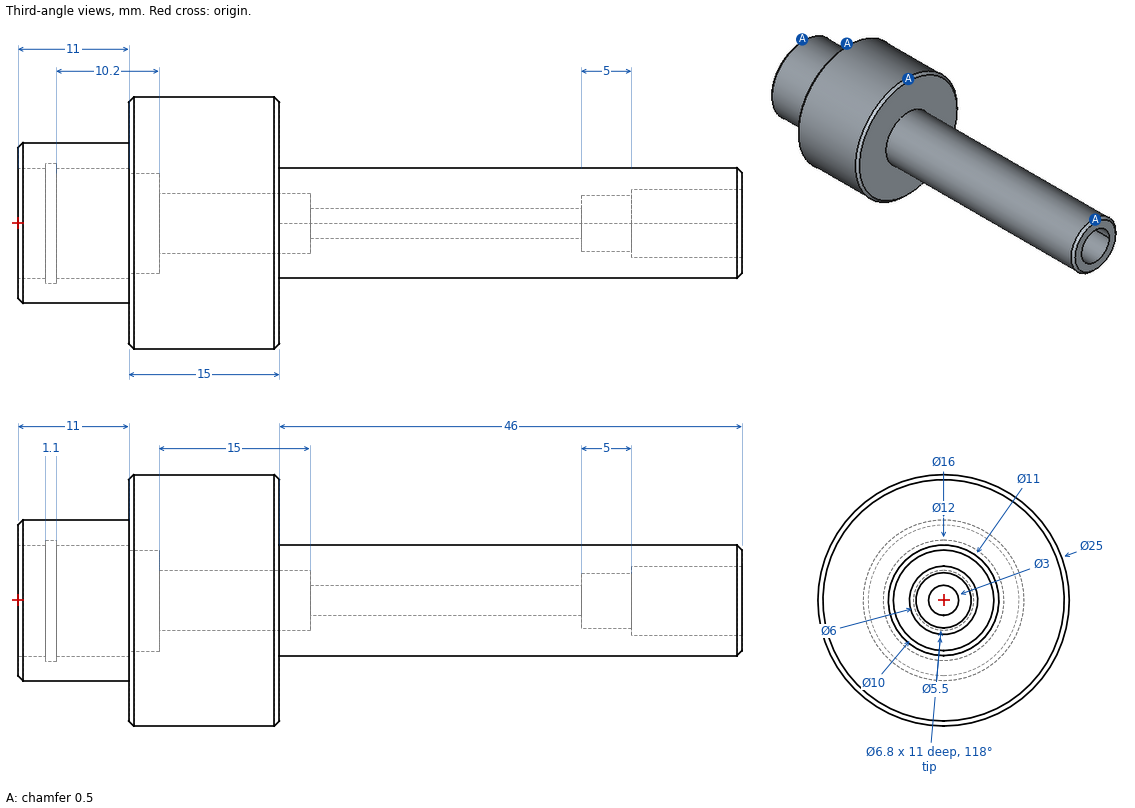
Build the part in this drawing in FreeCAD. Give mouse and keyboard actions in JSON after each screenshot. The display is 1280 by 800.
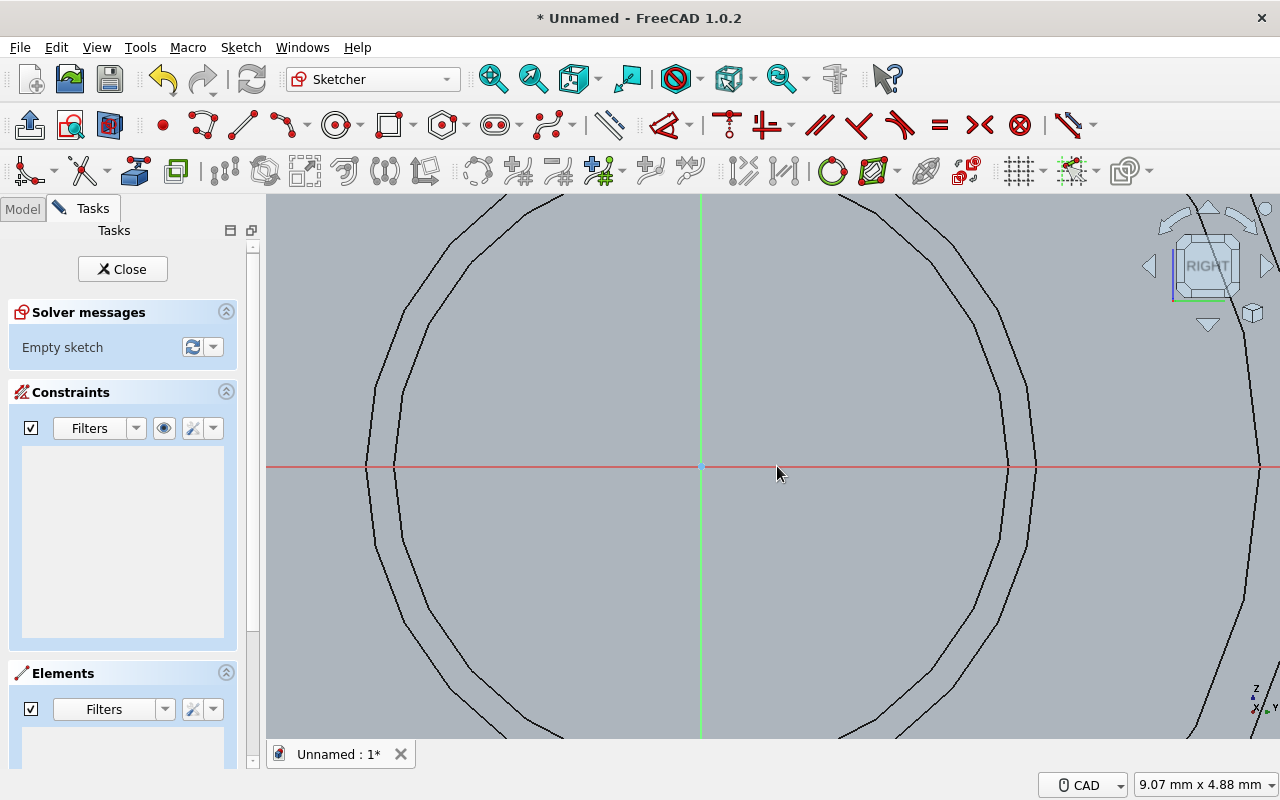
{"action": "left_click", "coordinate": [336, 126]}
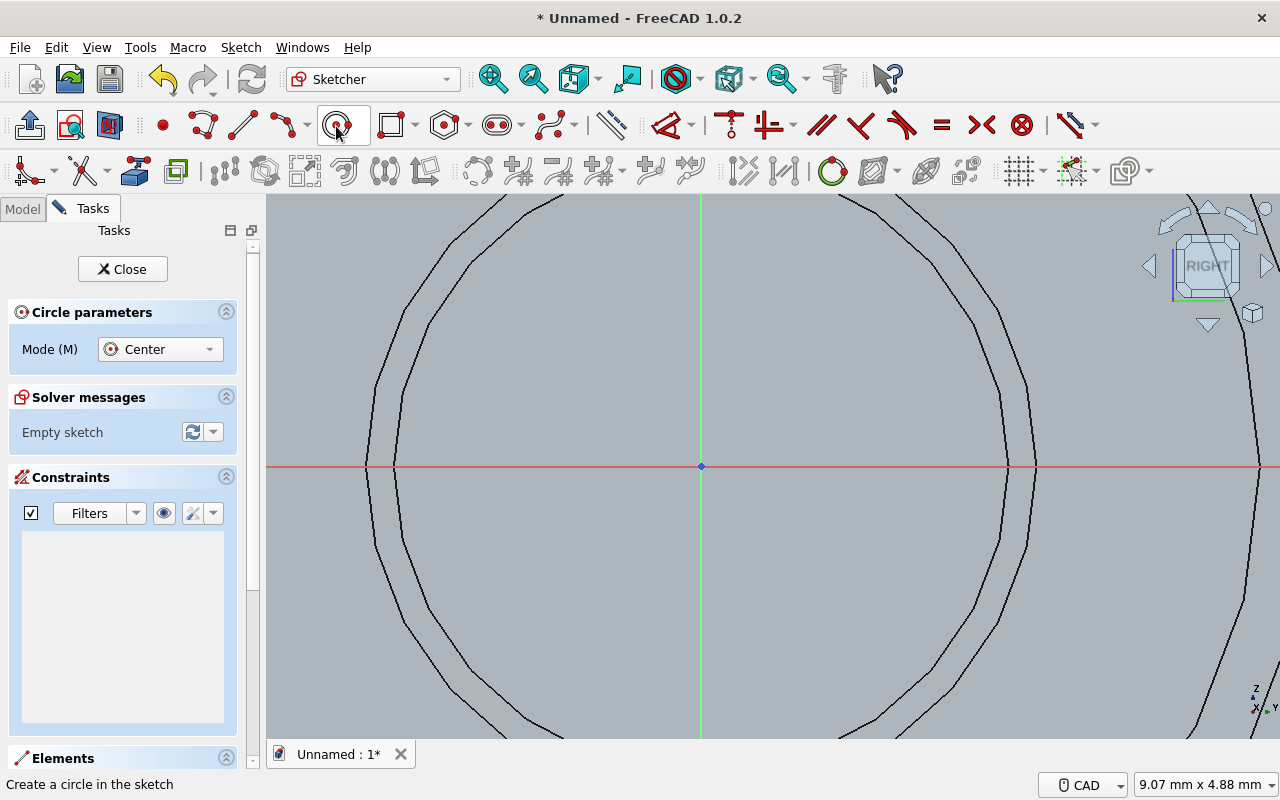
{"action": "left_click", "coordinate": [701, 466]}
{"action": "mouse_move", "coordinate": [820, 348]}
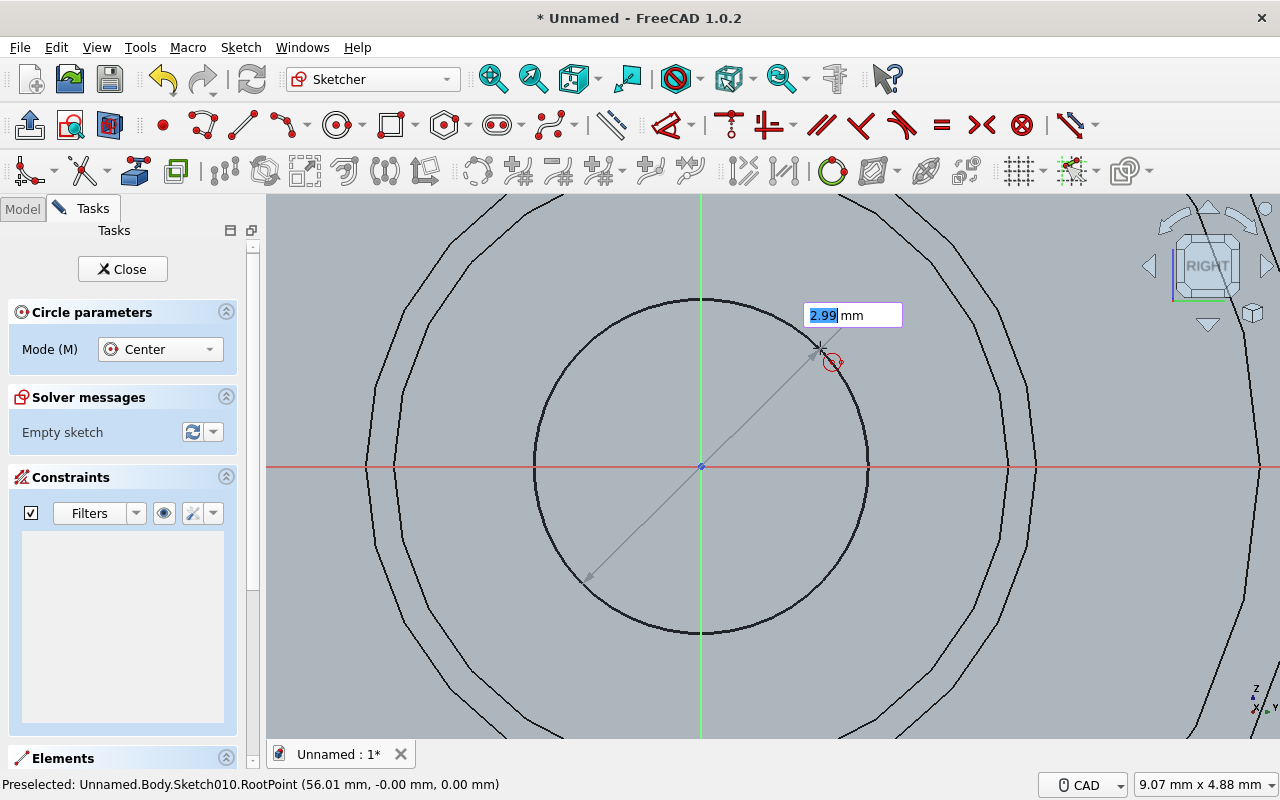
{"action": "type", "text": "3"}
{"action": "key", "text": "Return"}
{"action": "key", "text": "Escape"}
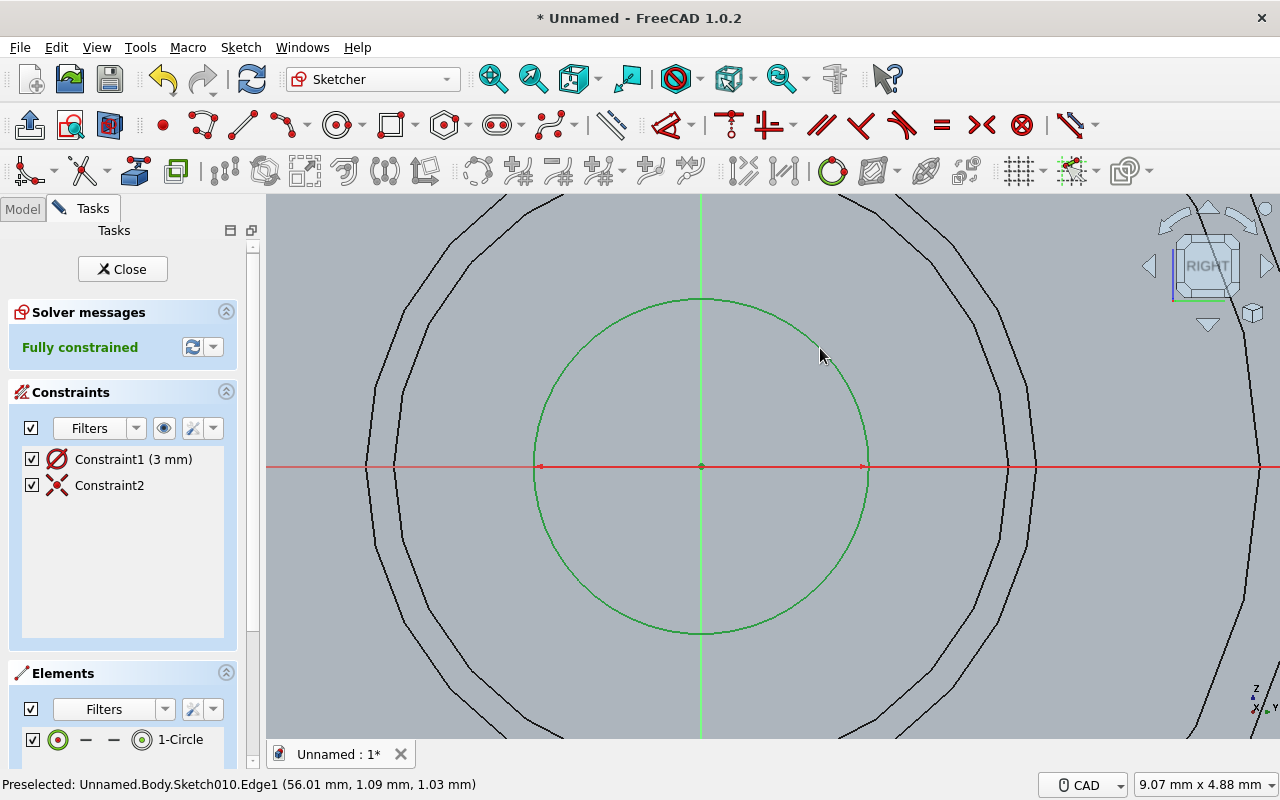
{"action": "left_click", "coordinate": [123, 269]}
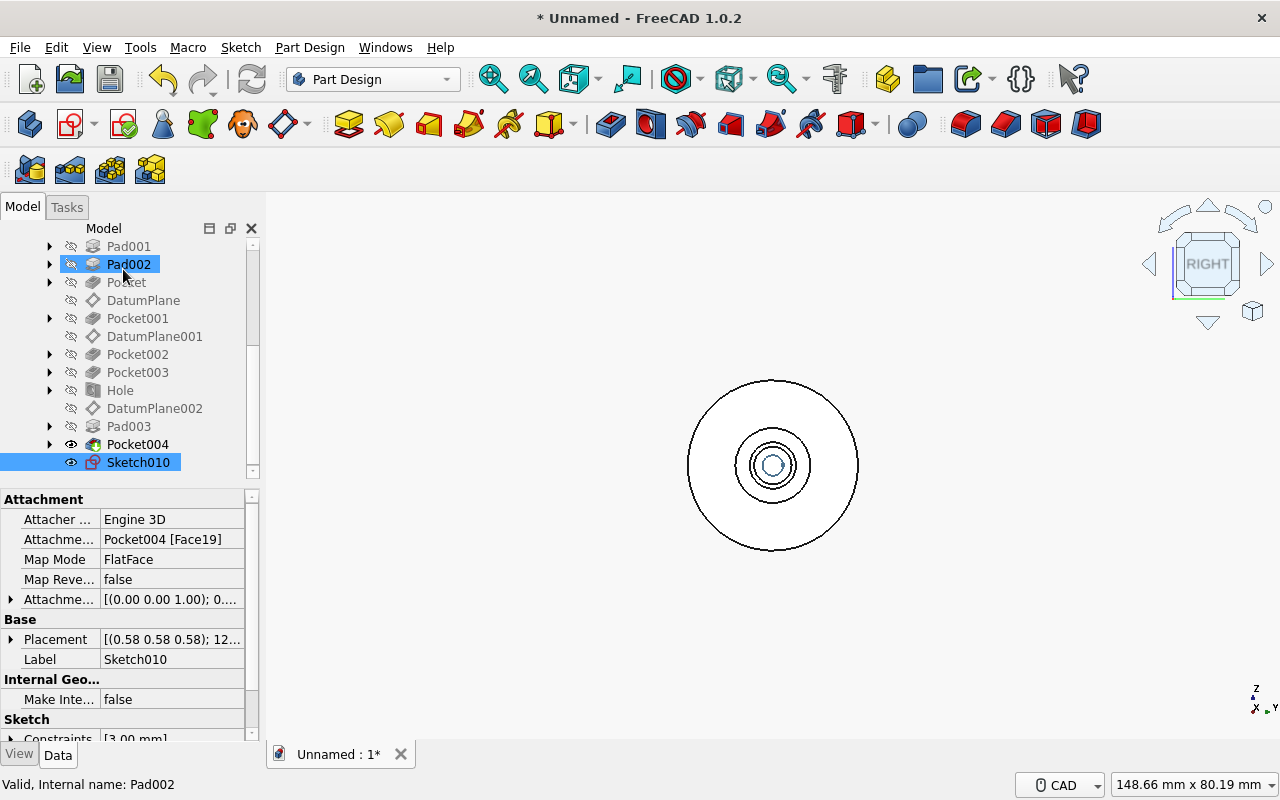
{"action": "left_click", "coordinate": [612, 124]}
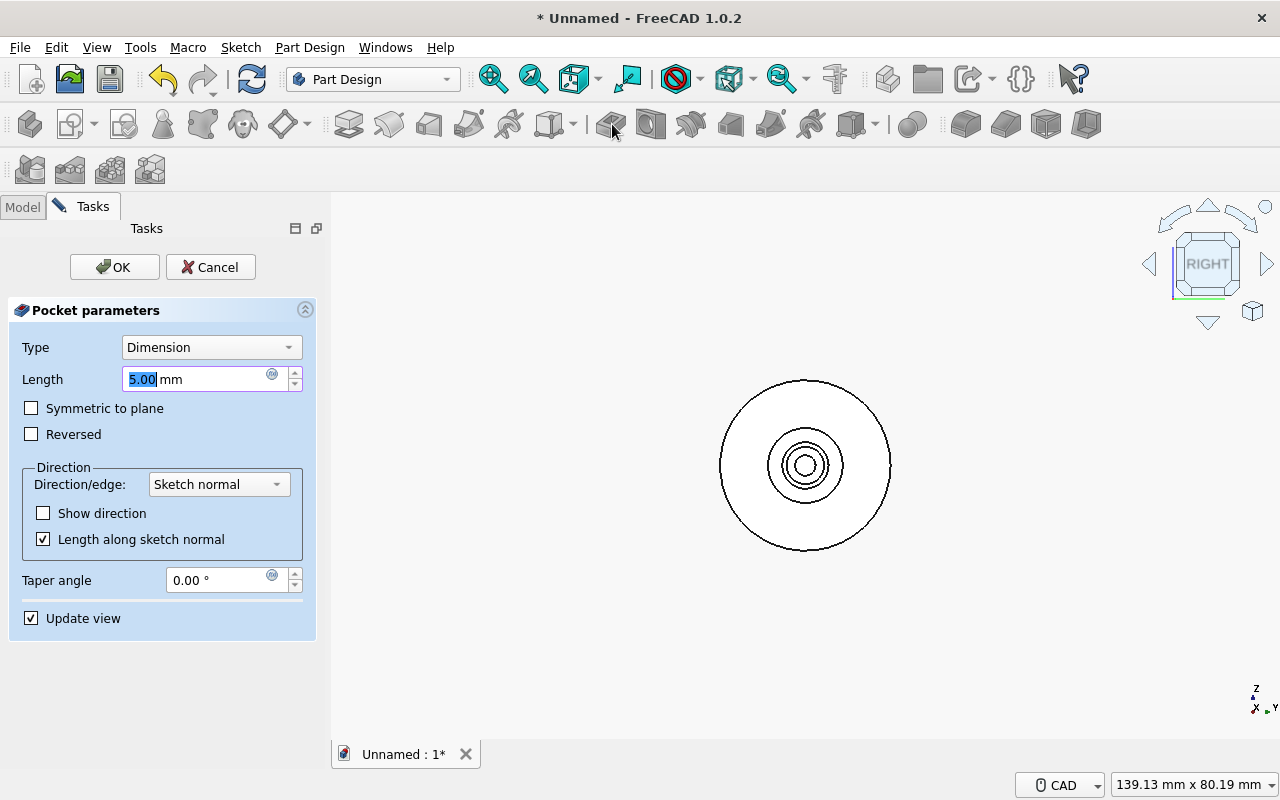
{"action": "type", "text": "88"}
{"action": "key", "text": "Tab"}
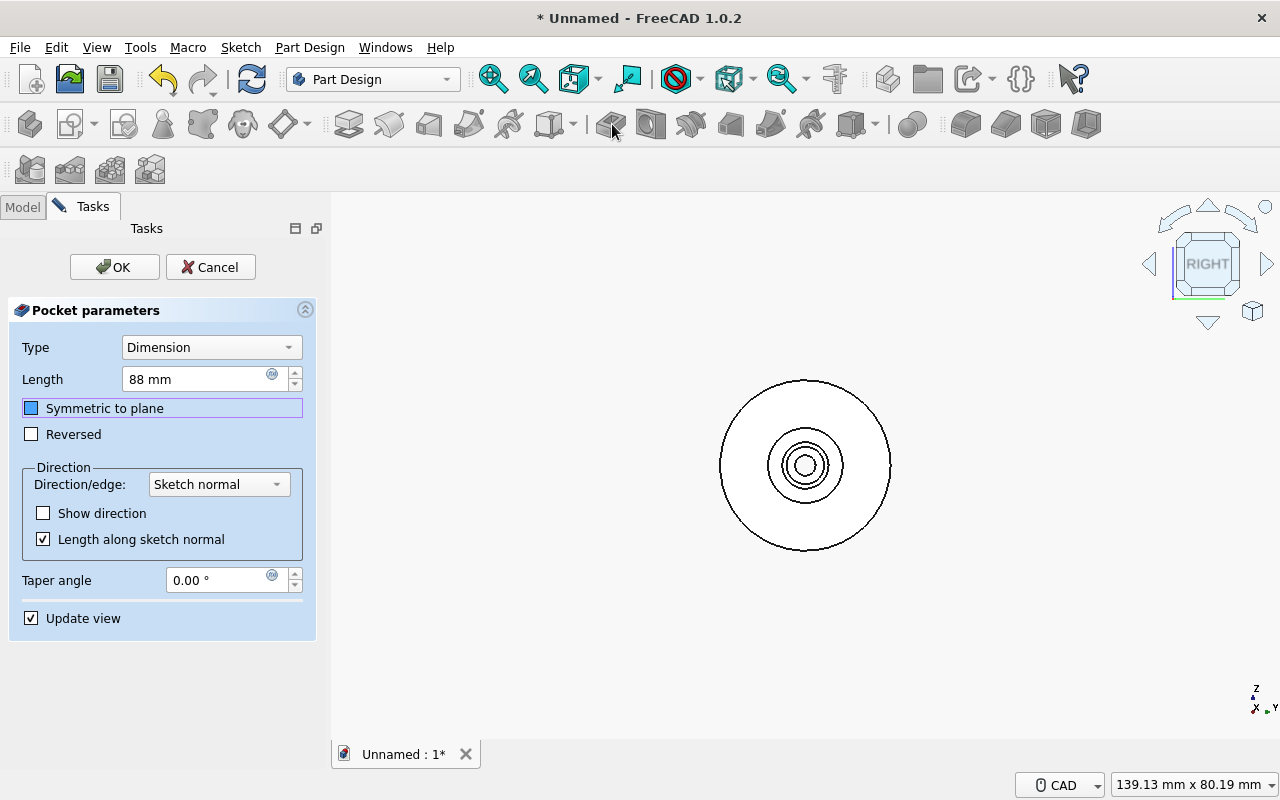
{"action": "left_click", "coordinate": [115, 267]}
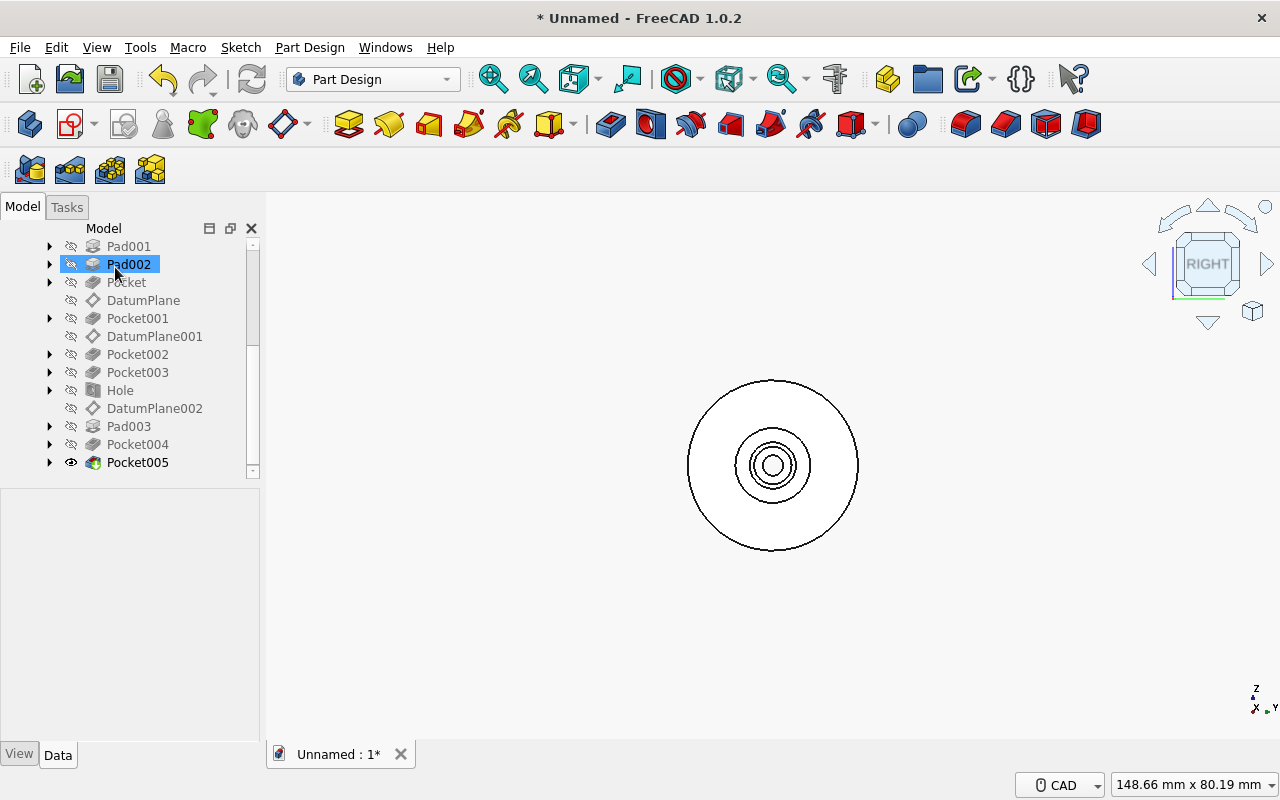
{"action": "left_click", "coordinate": [494, 80]}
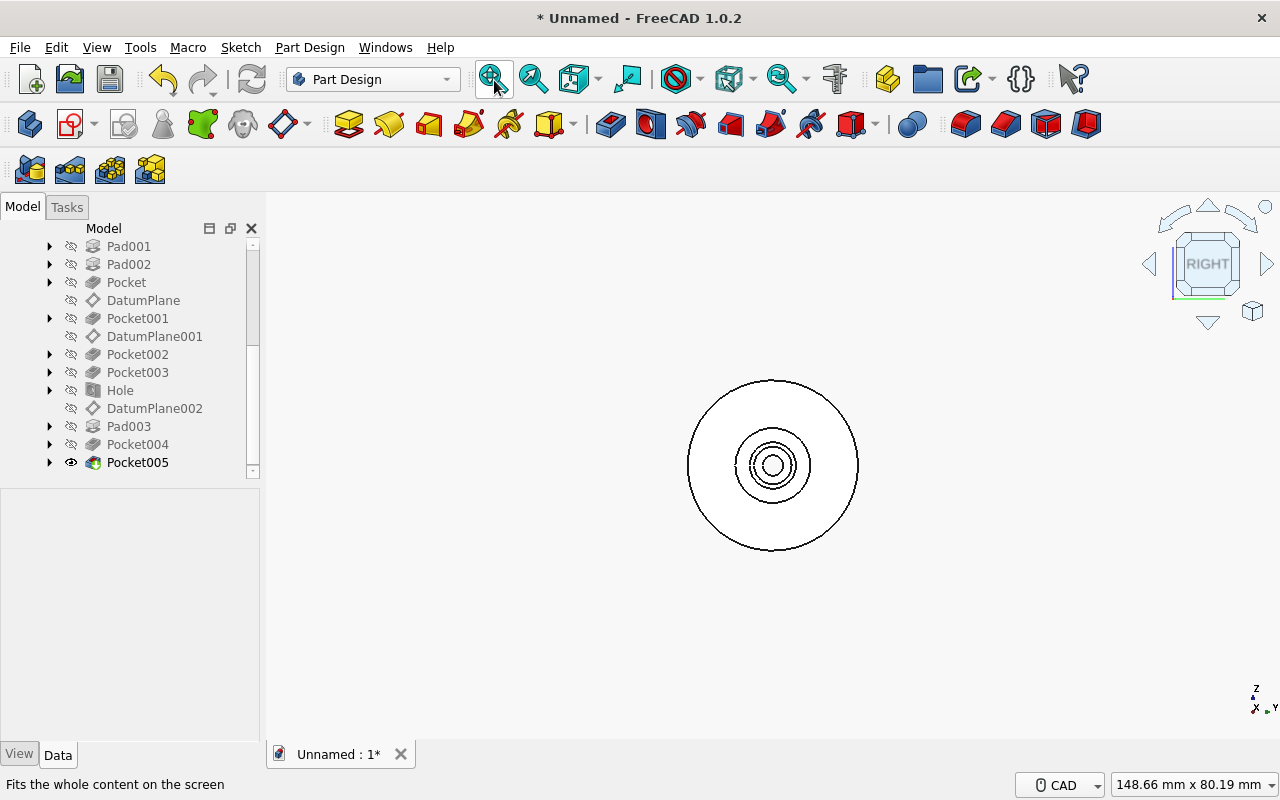
{"action": "left_click", "coordinate": [743, 487]}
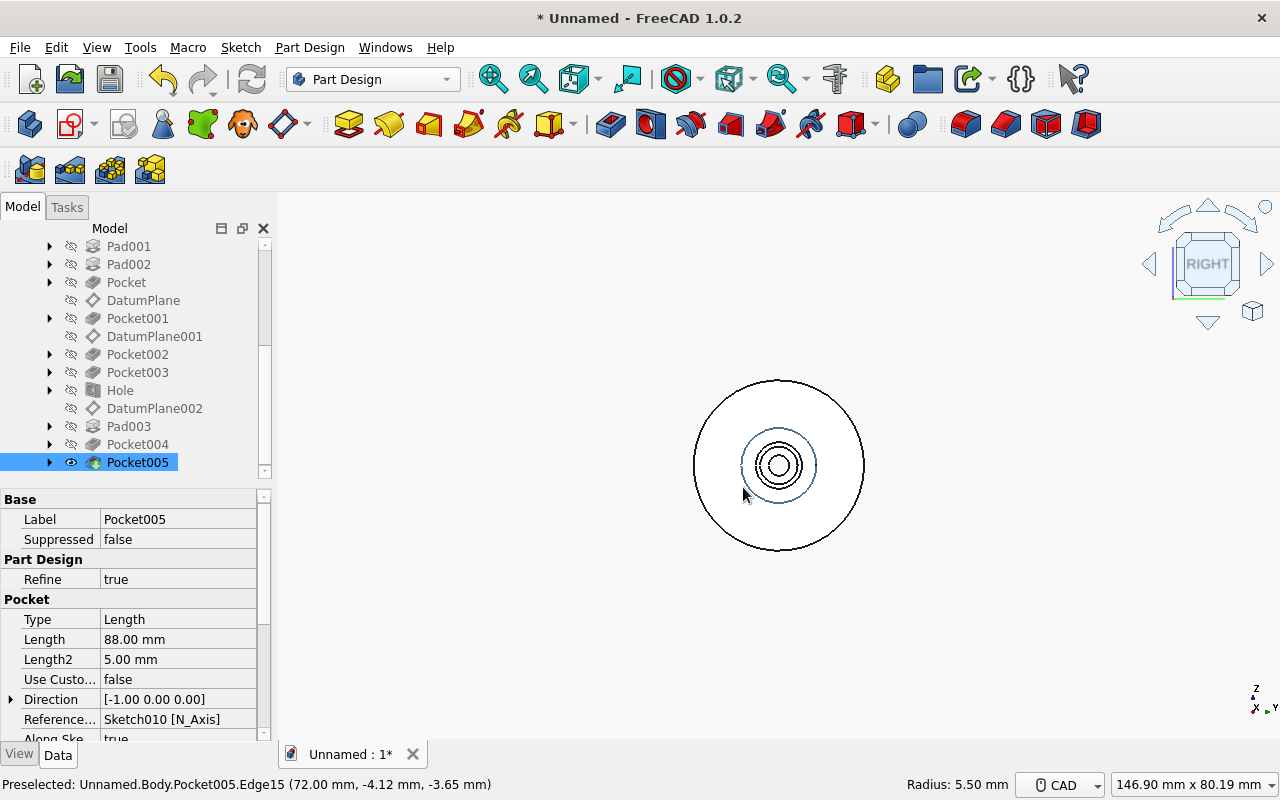
{"action": "left_click", "coordinate": [753, 546], "text": "ctrl"}